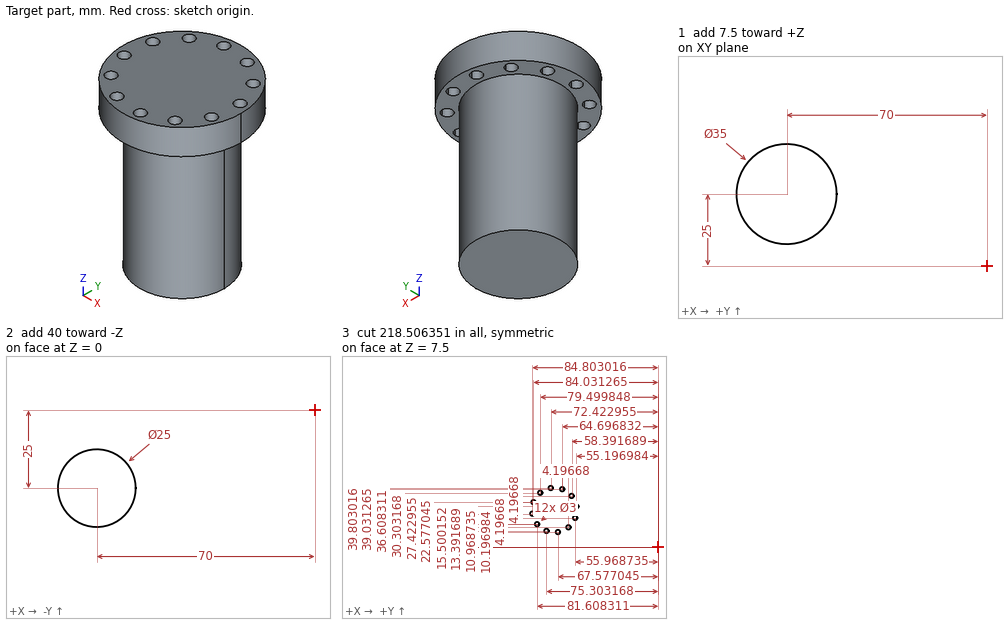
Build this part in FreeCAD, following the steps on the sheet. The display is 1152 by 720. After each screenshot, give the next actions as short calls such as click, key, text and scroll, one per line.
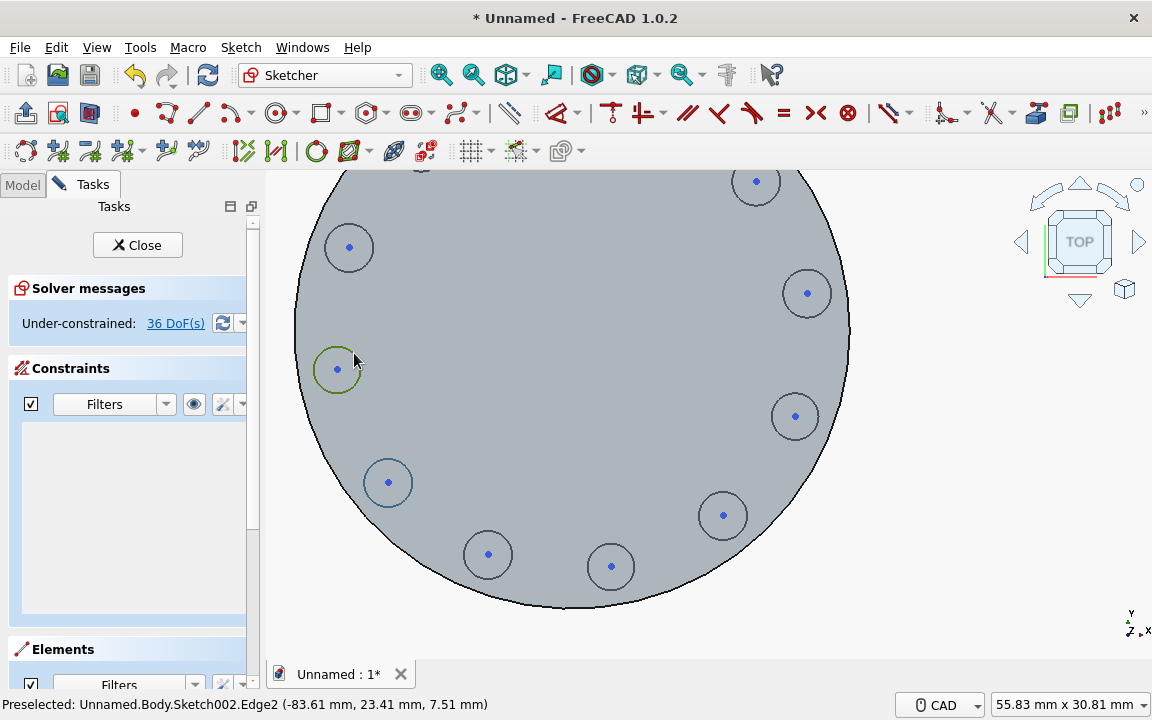
click(366, 231)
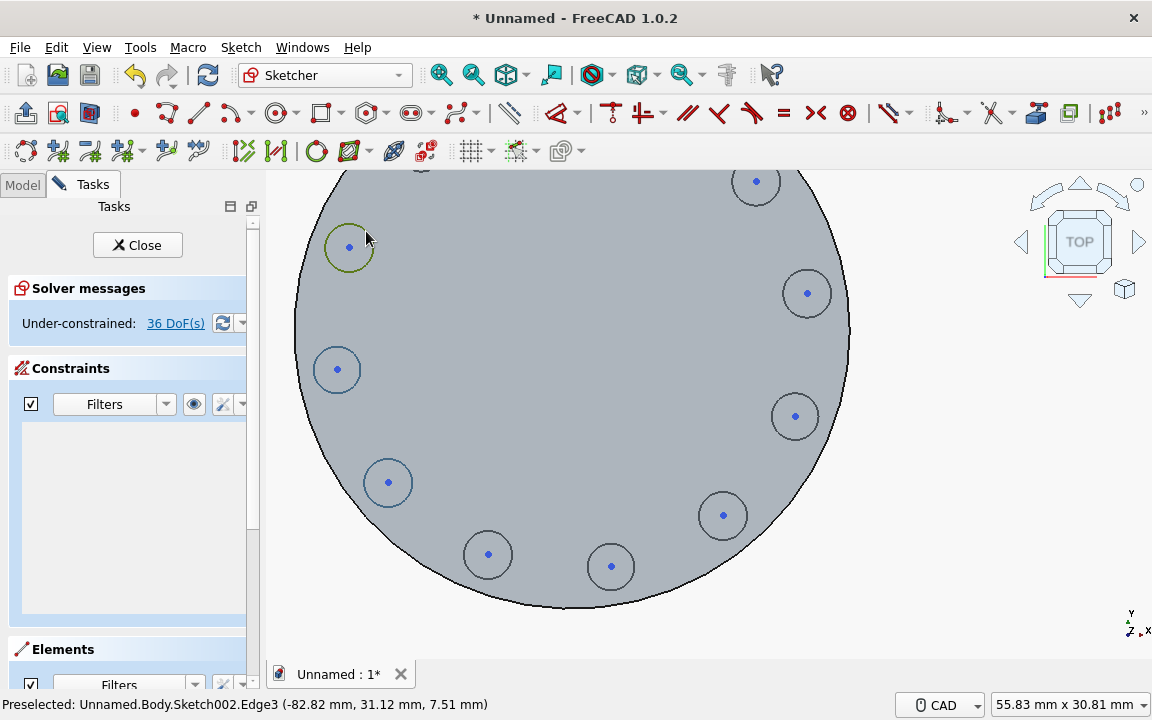
scroll(724, 516, down, 3)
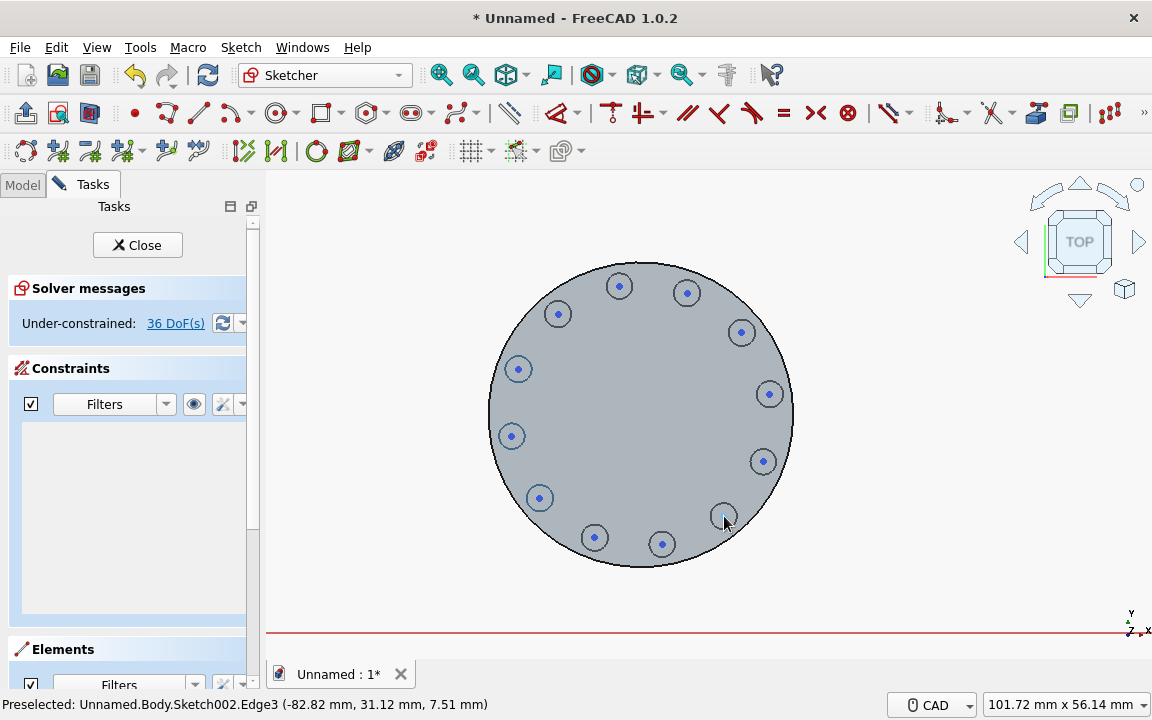
click(567, 305)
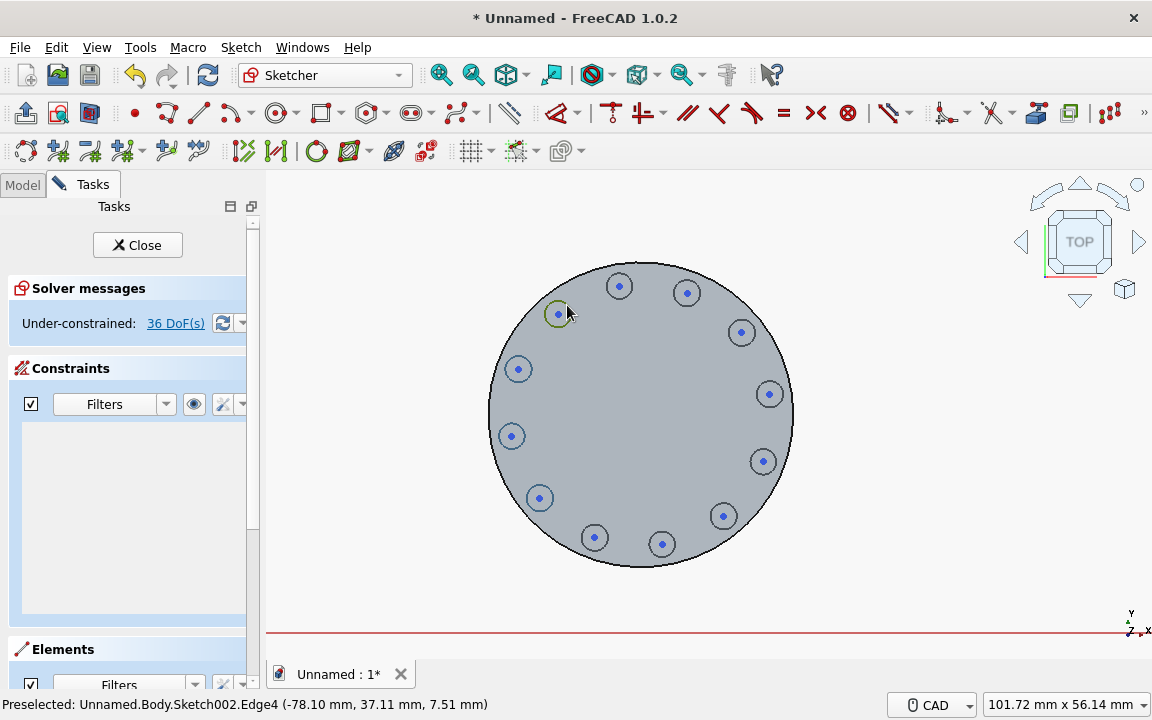
click(629, 277)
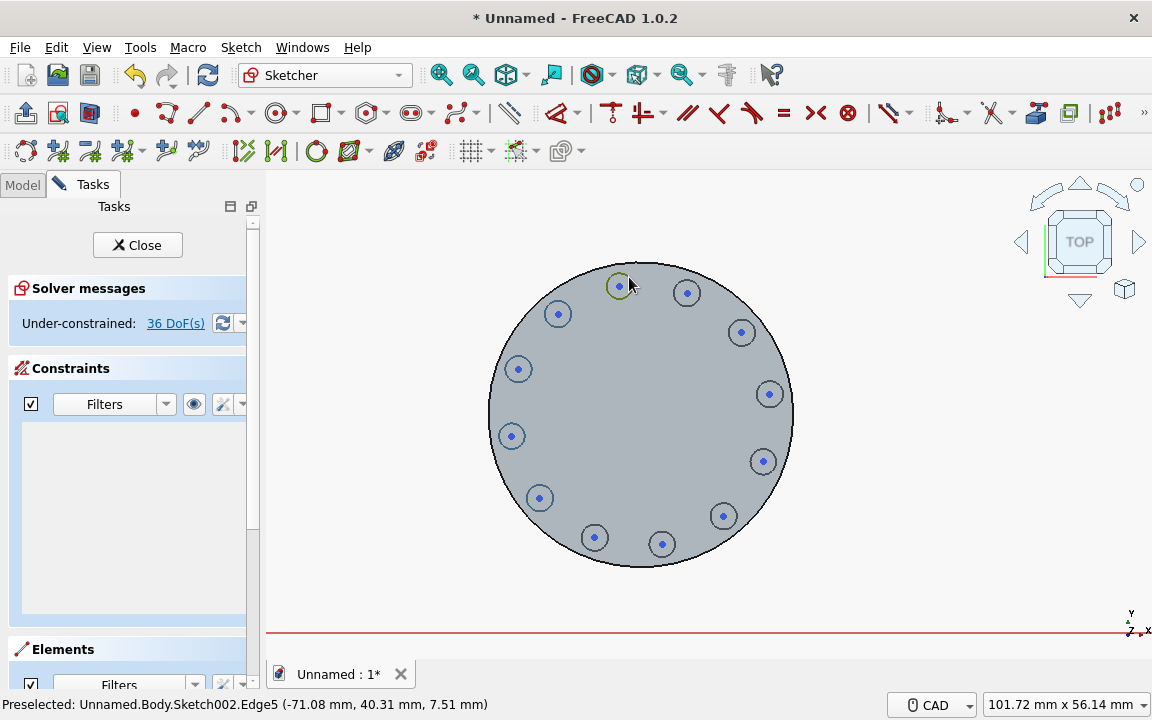
click(696, 284)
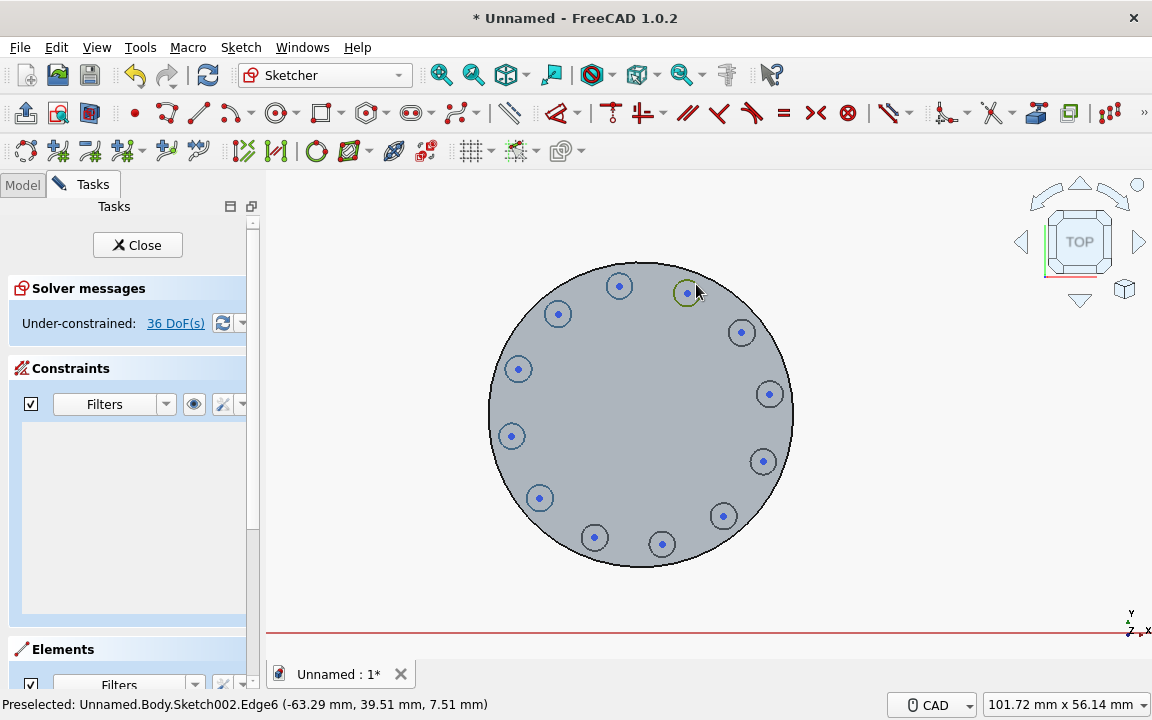
click(751, 323)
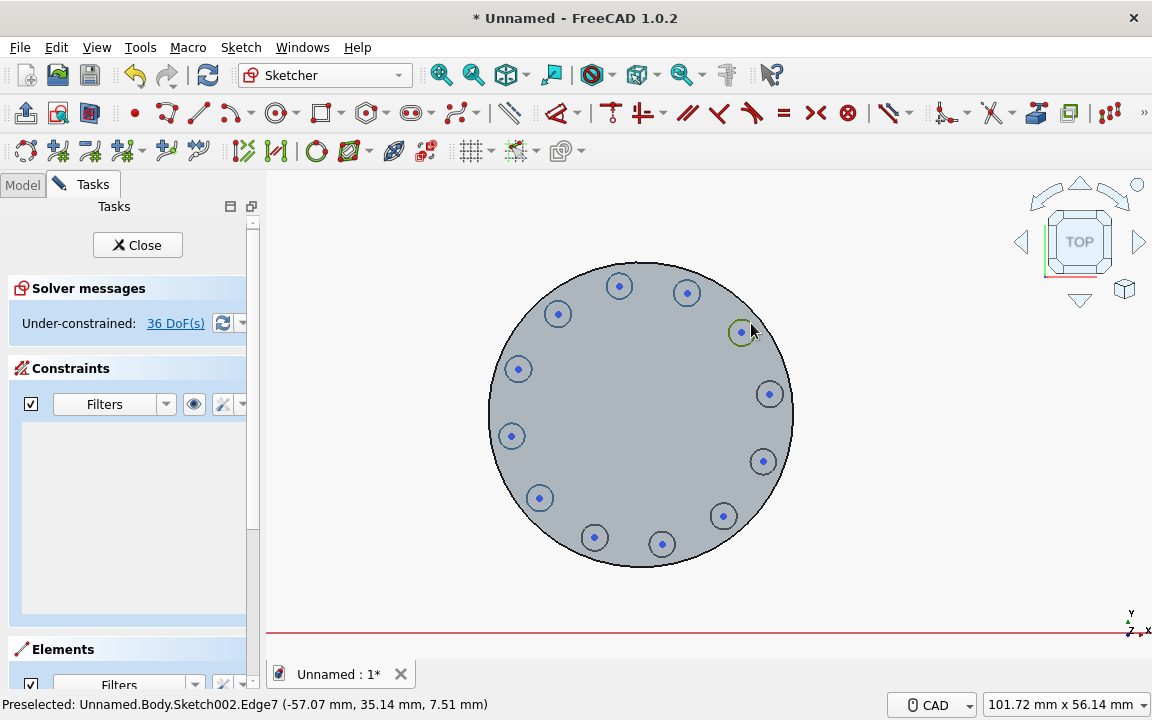
click(779, 385)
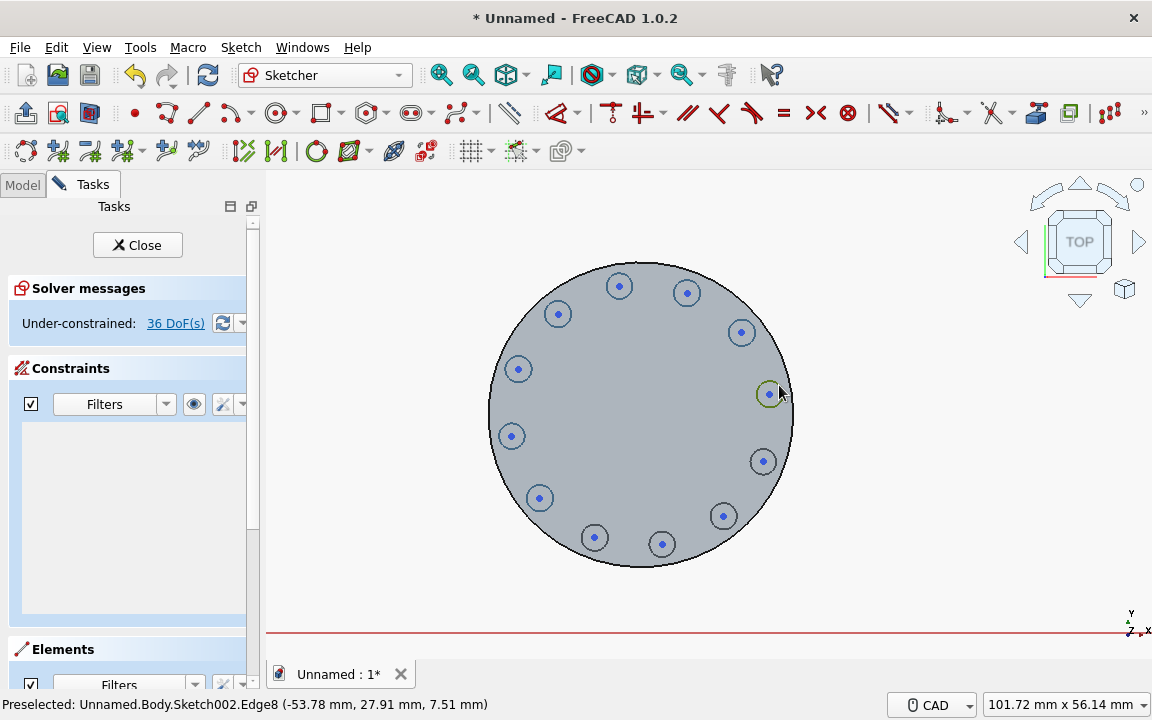
click(772, 453)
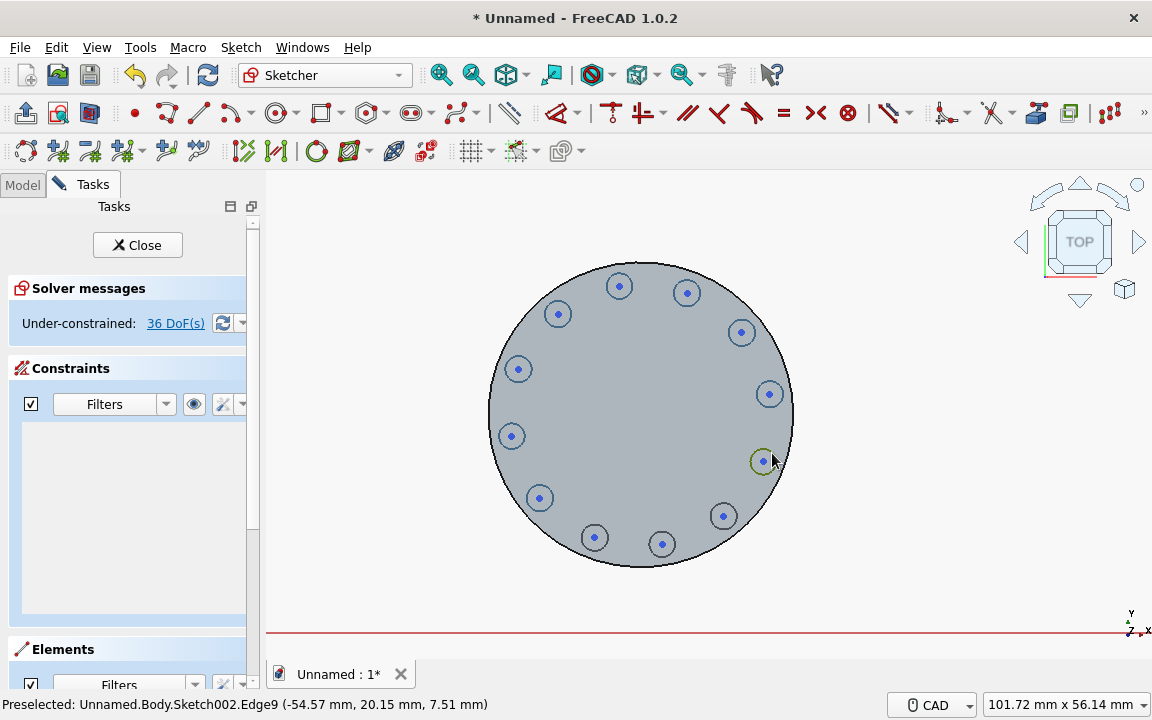
click(733, 507)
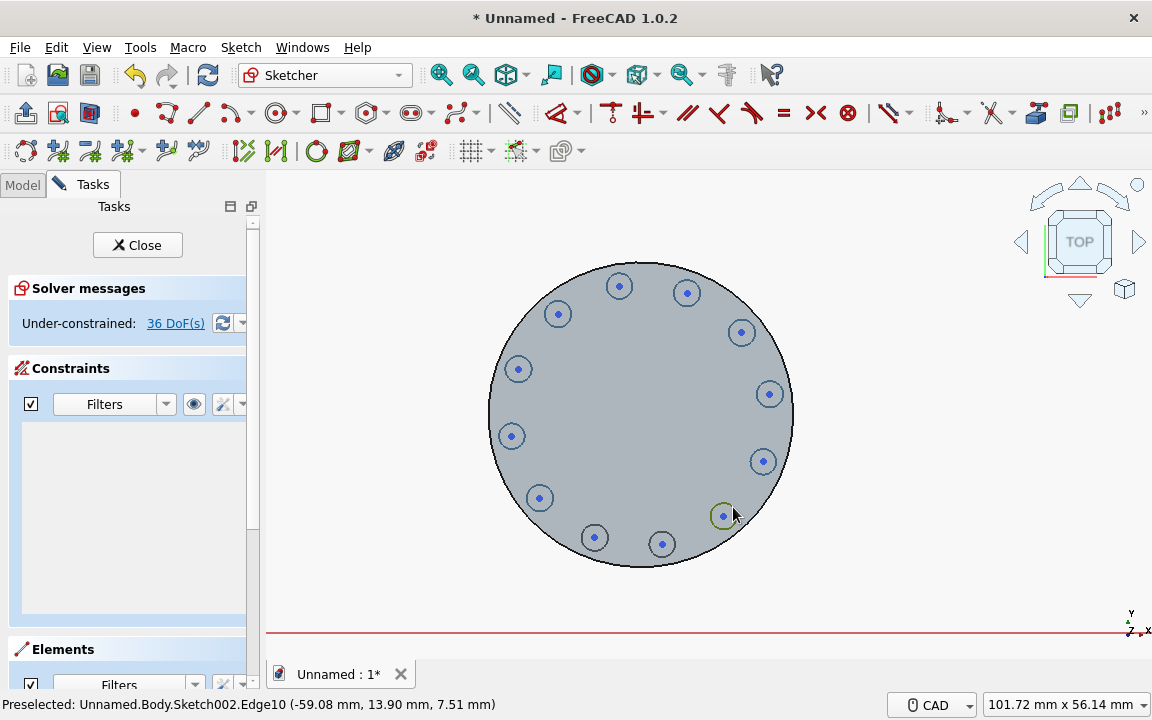
click(671, 535)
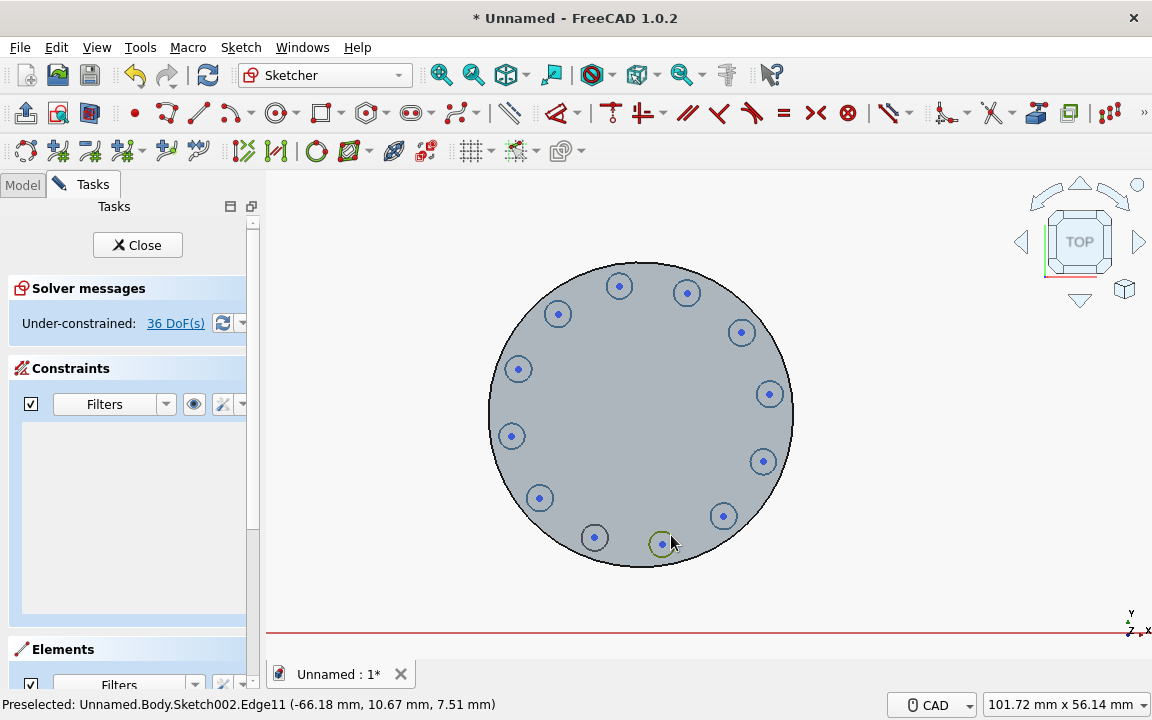
click(604, 528)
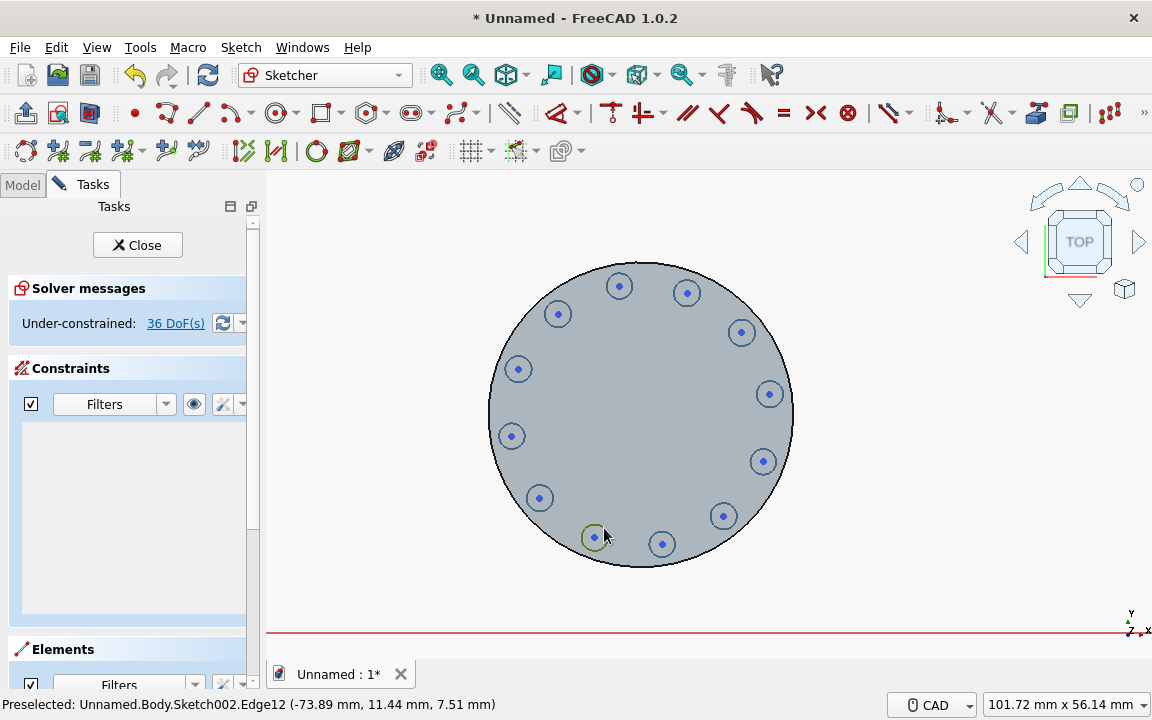
key(e)